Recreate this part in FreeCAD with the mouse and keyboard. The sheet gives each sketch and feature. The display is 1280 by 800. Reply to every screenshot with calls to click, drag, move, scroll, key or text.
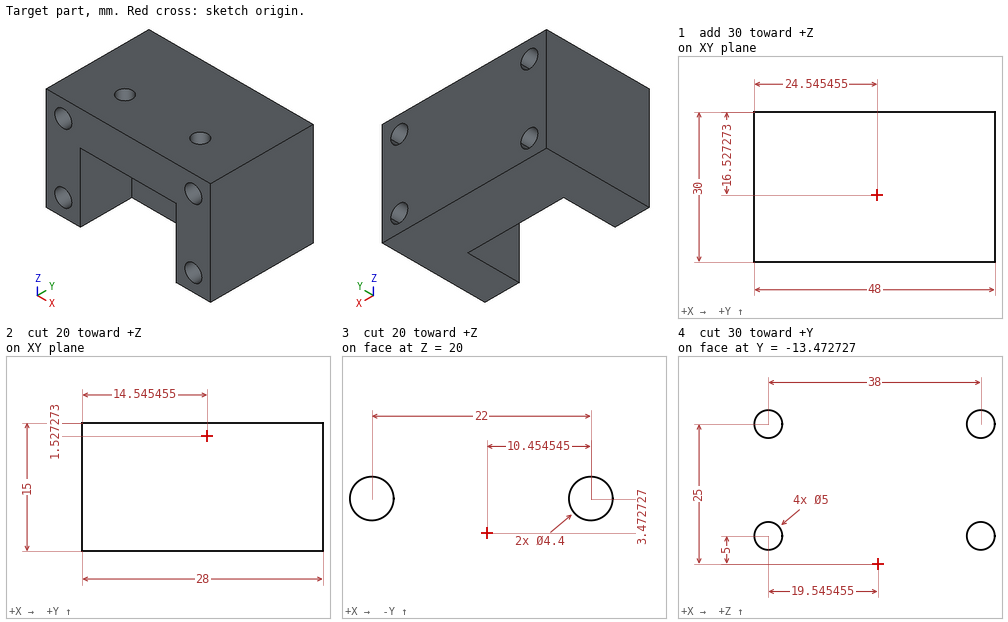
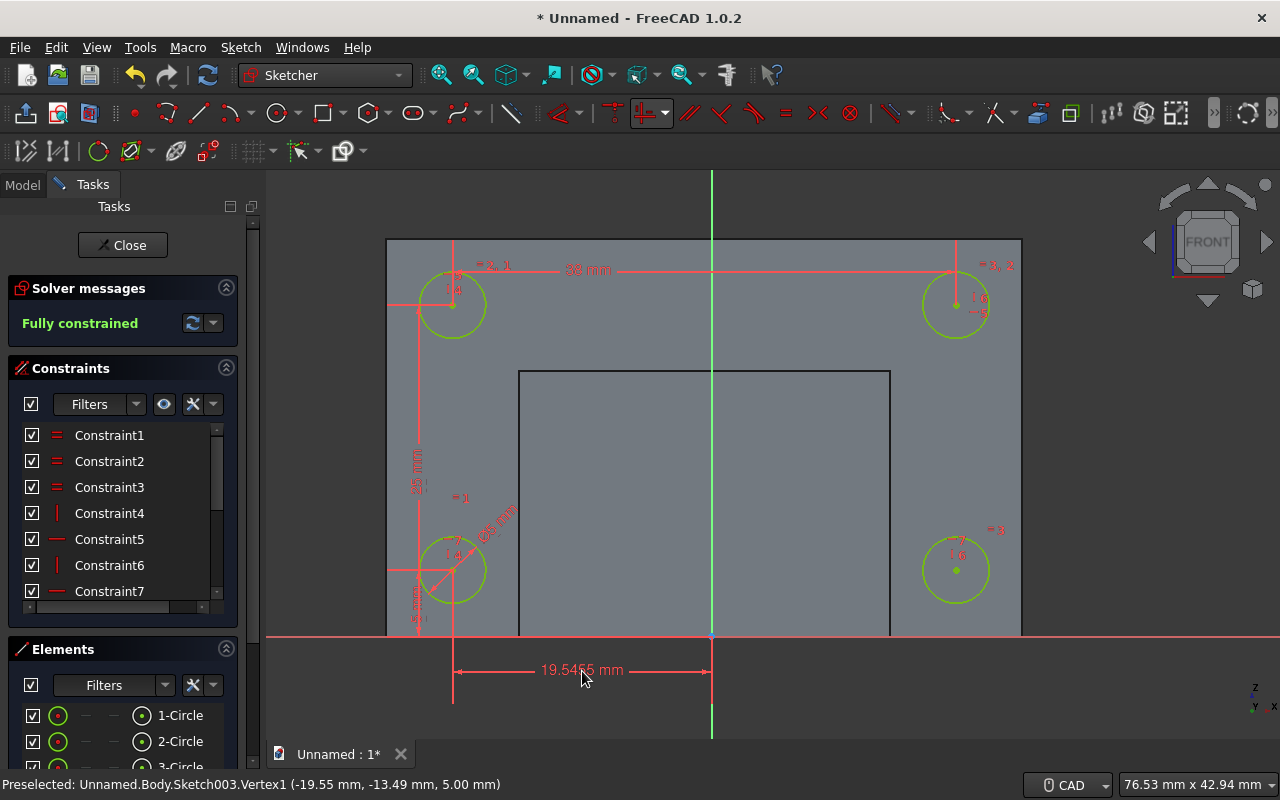
click(123, 245)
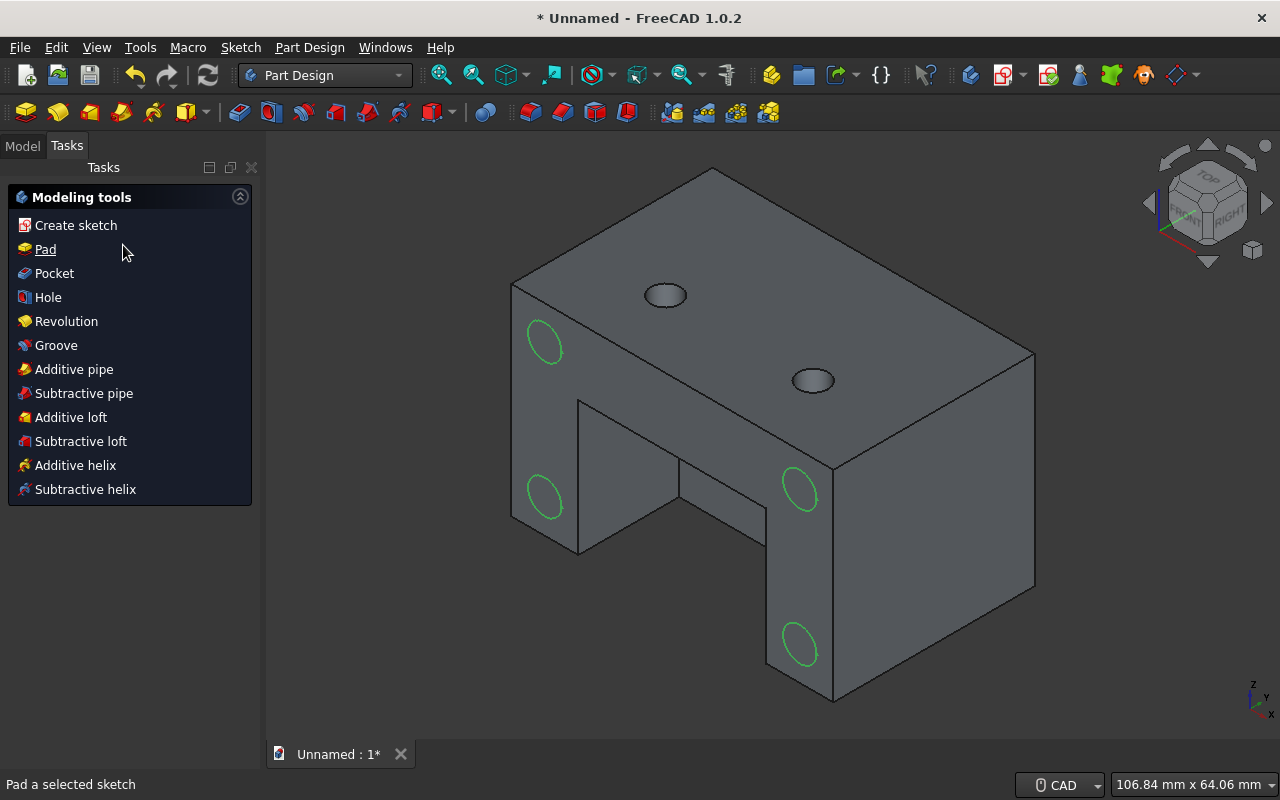
click(240, 112)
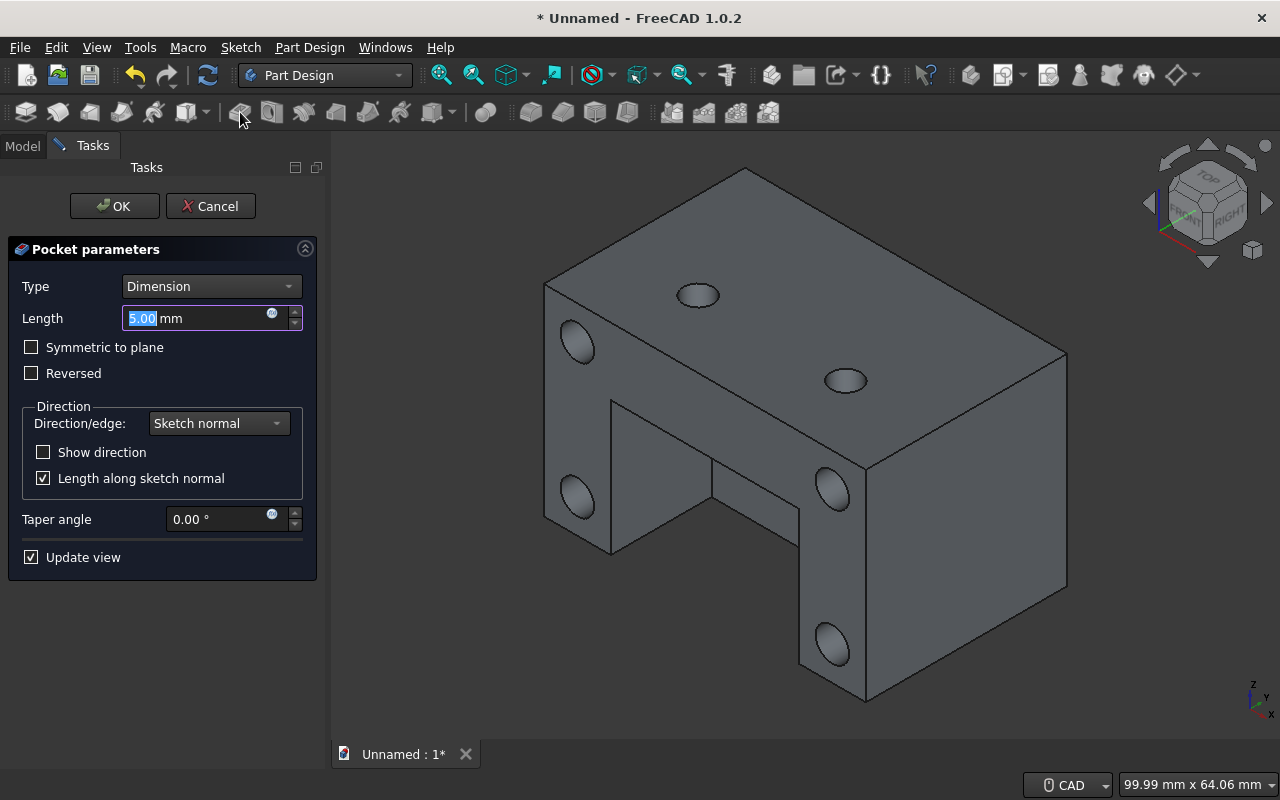
text(30)
key(Tab)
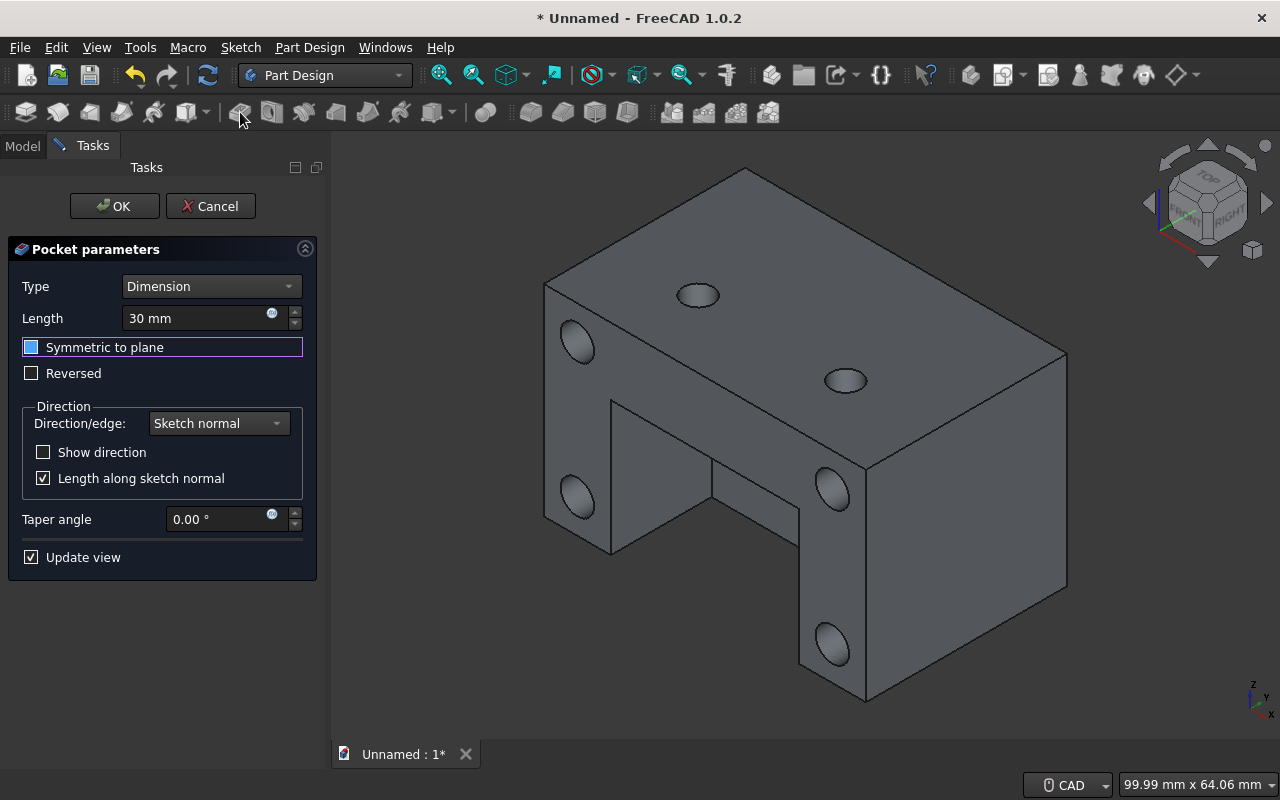
click(115, 206)